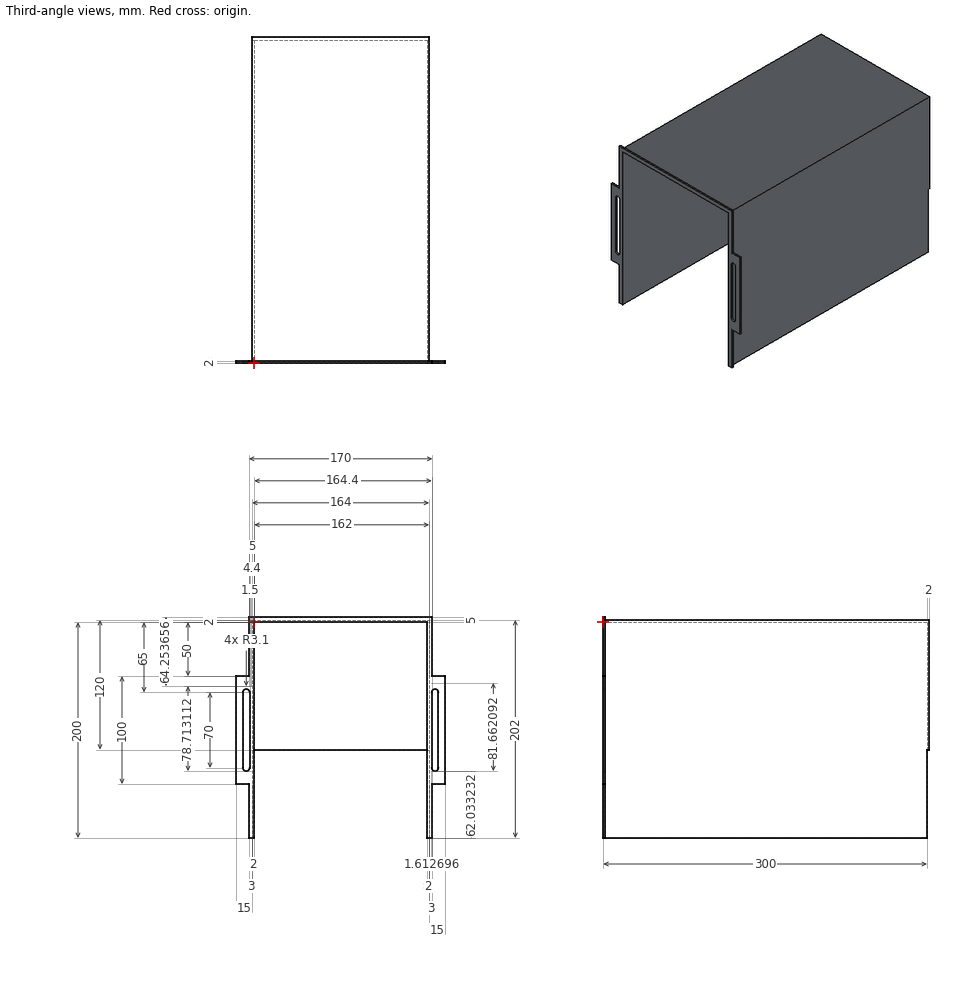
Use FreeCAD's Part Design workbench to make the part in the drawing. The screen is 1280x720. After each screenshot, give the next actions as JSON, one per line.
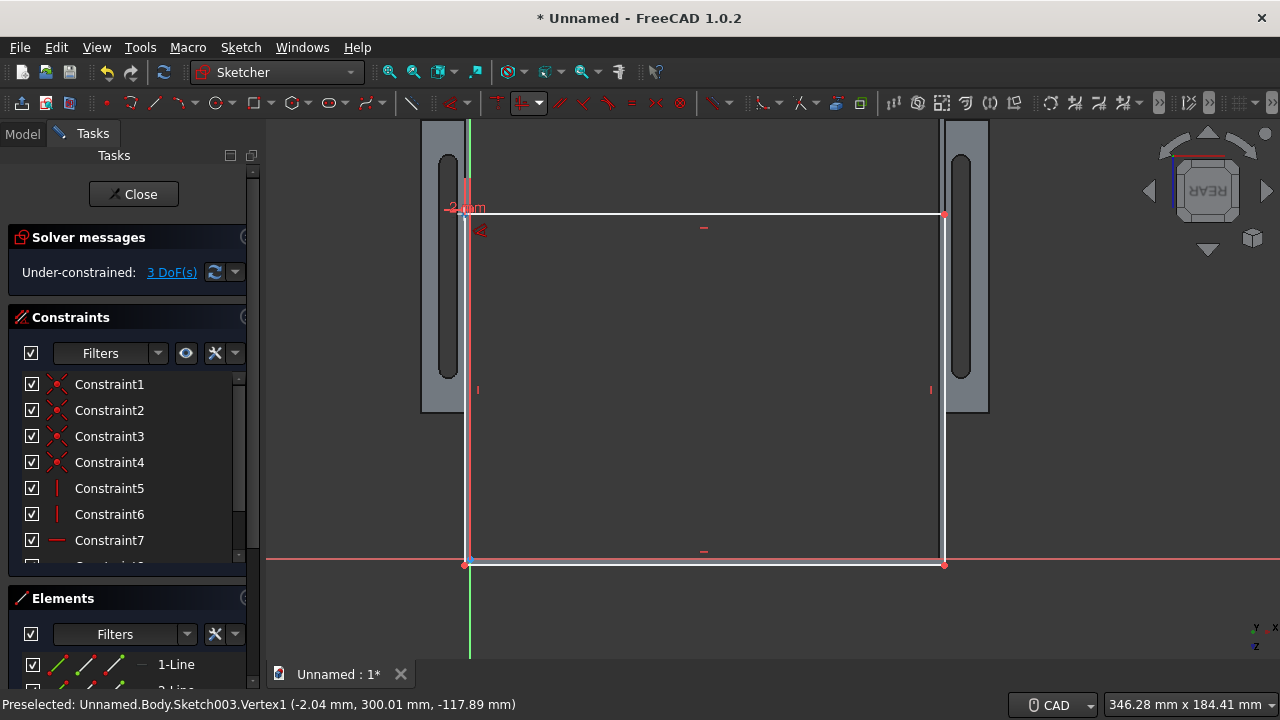
{"action": "scroll", "coordinate": [465, 565], "scroll_direction": "up", "scroll_amount": 10}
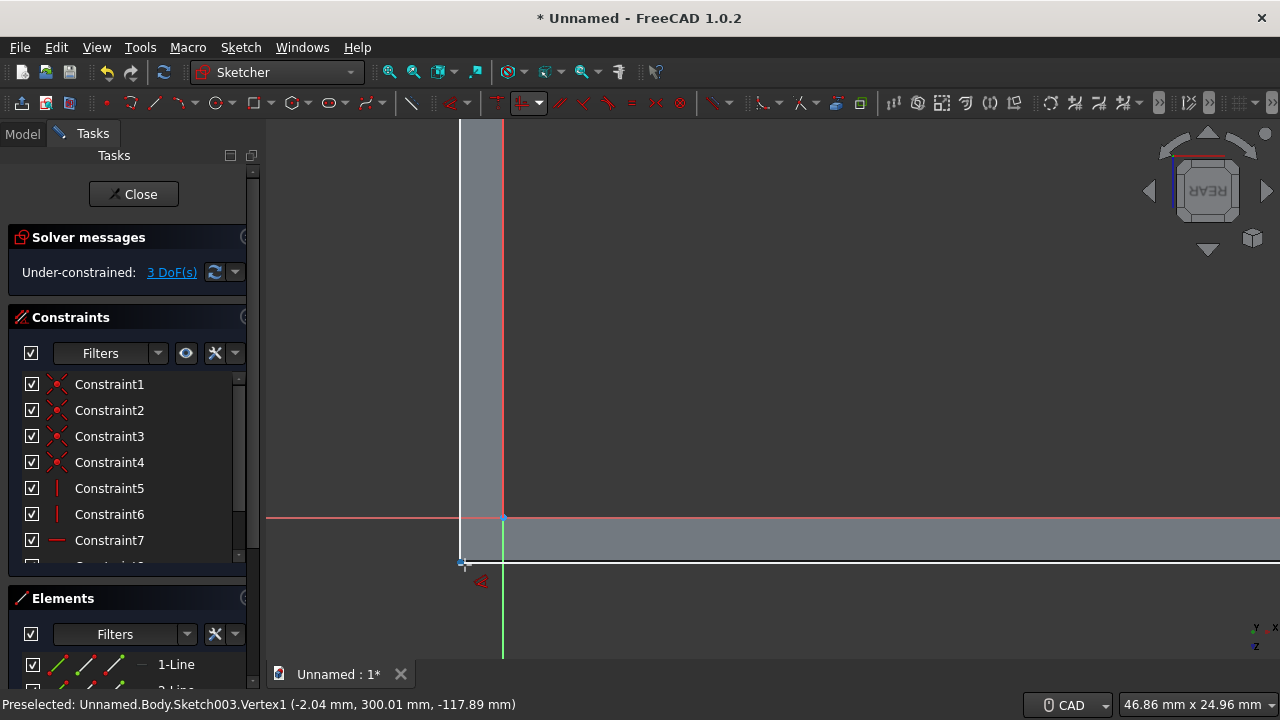
{"action": "left_click", "coordinate": [460, 563]}
{"action": "left_click", "coordinate": [426, 540]}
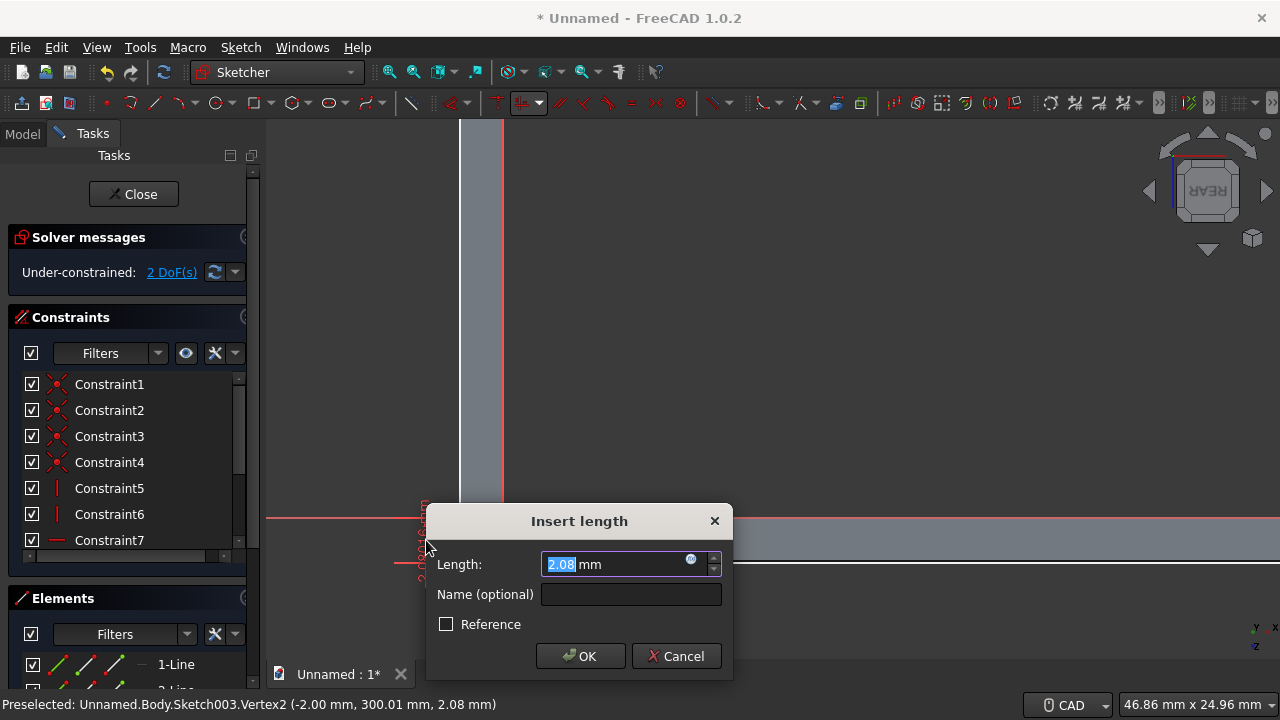
{"action": "type", "text": "2"}
{"action": "key", "text": "Return"}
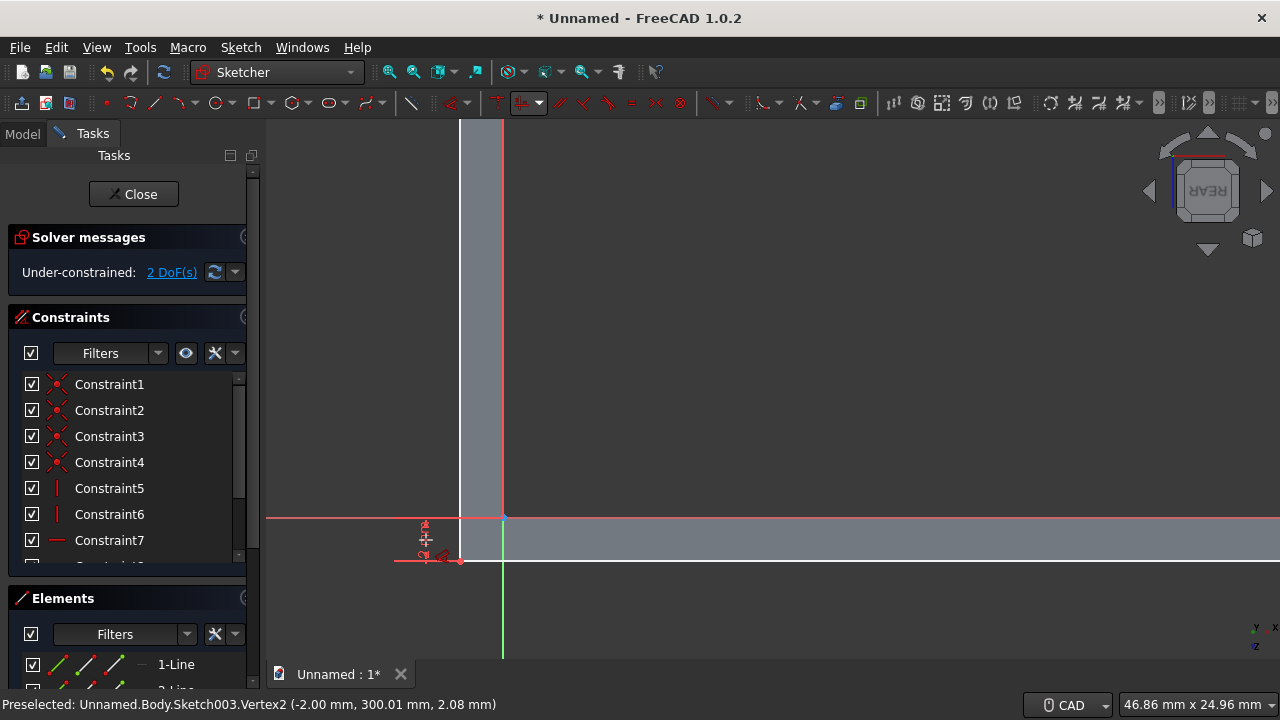
{"action": "scroll", "coordinate": [465, 565], "scroll_direction": "down", "scroll_amount": 10}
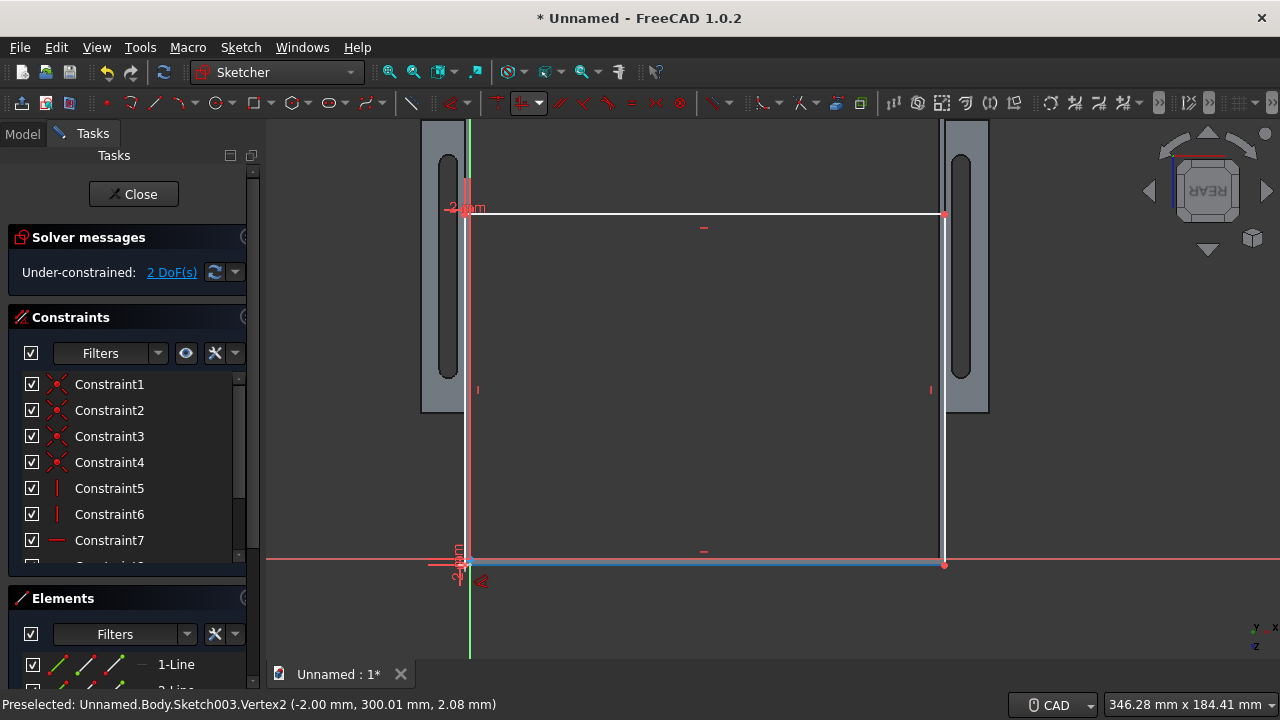
{"action": "scroll", "coordinate": [465, 319], "scroll_direction": "up", "scroll_amount": 5}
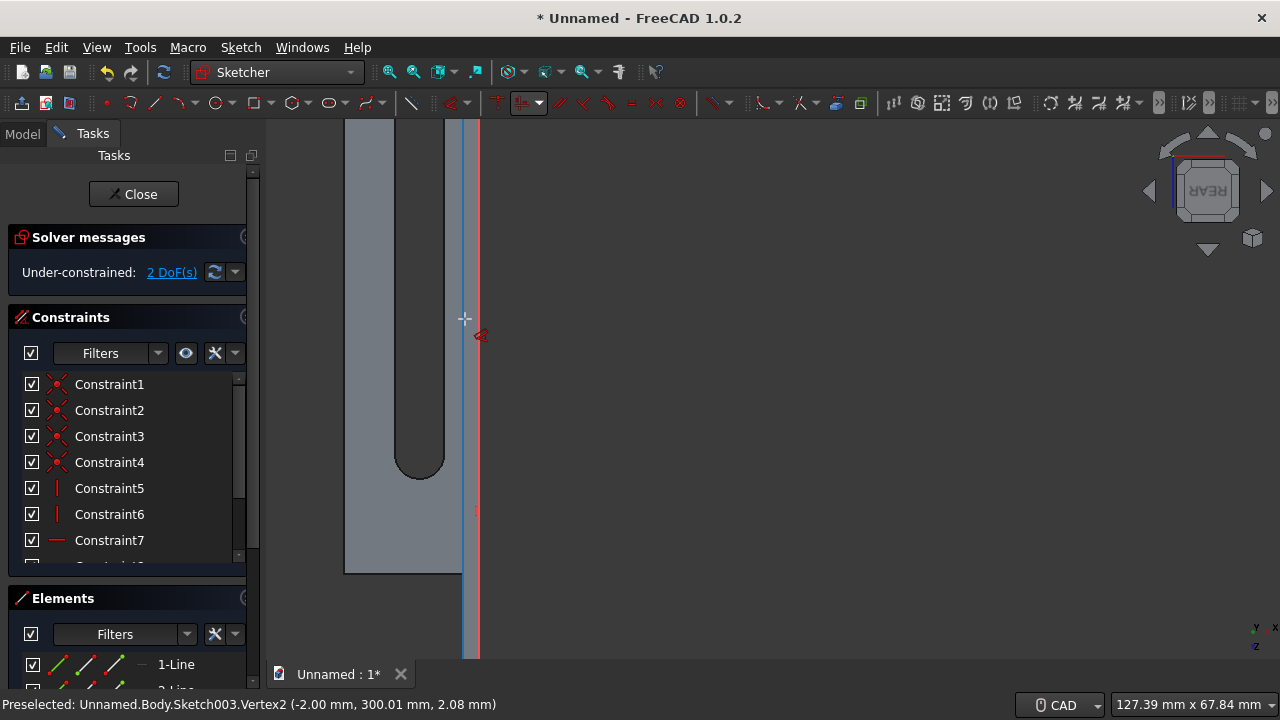
{"action": "left_click", "coordinate": [463, 320]}
{"action": "left_click", "coordinate": [429, 389]}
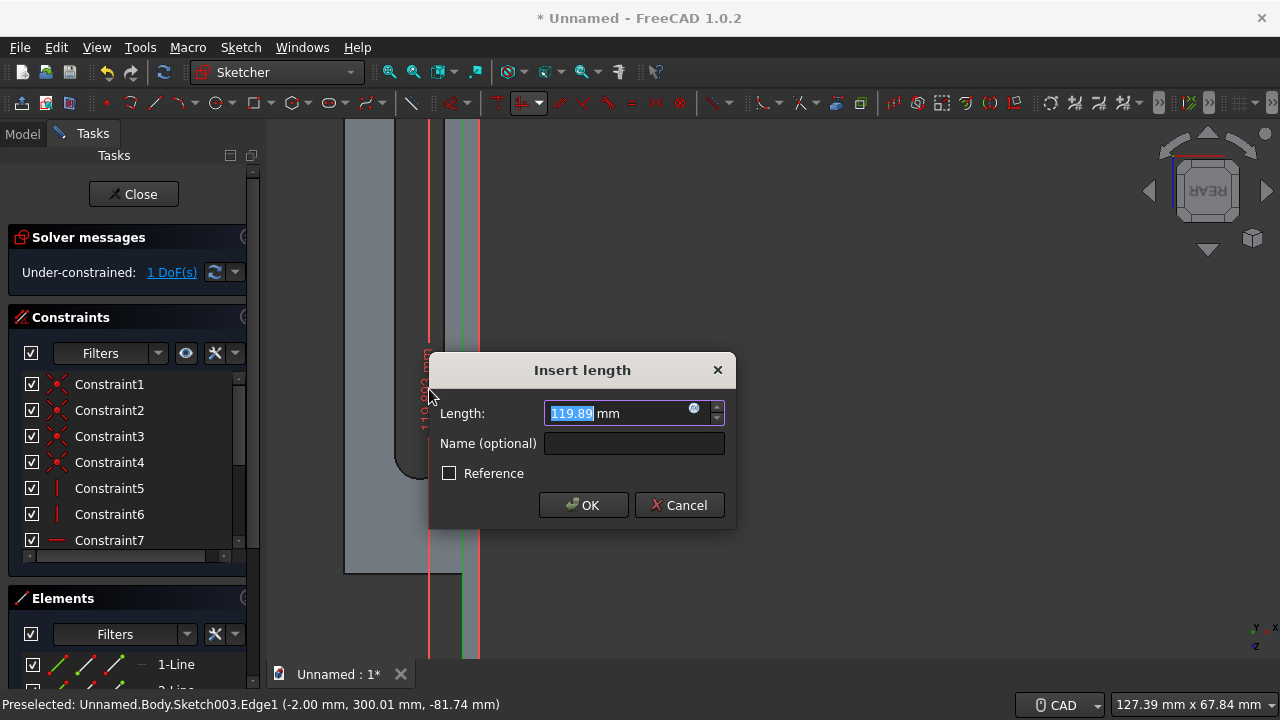
{"action": "type", "text": "120"}
{"action": "key", "text": "Return"}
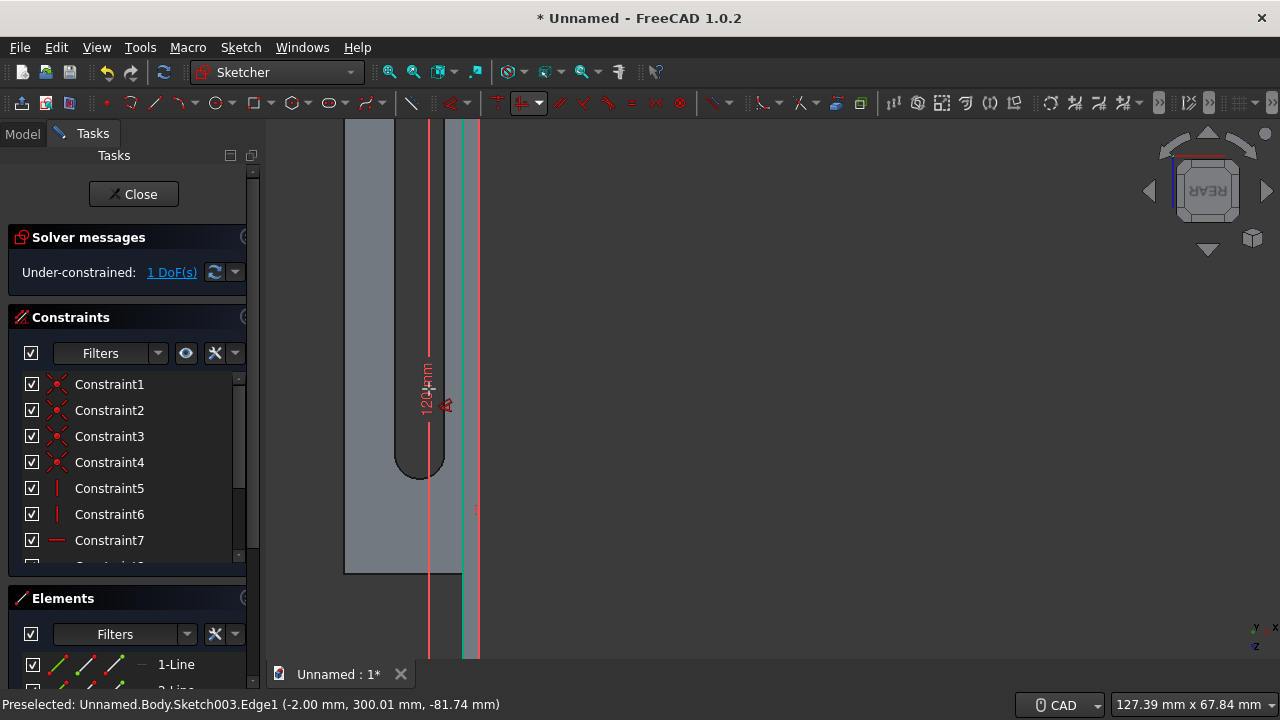
{"action": "scroll", "coordinate": [465, 319], "scroll_direction": "down", "scroll_amount": 5}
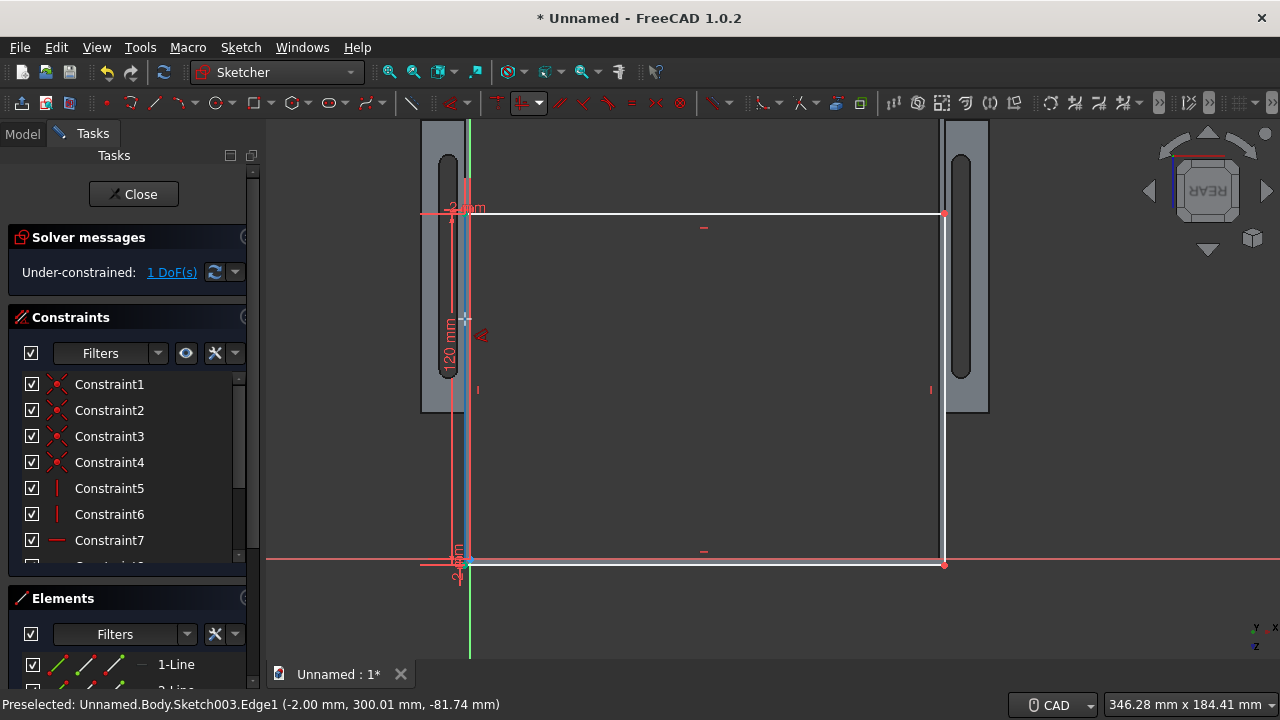
{"action": "scroll", "coordinate": [609, 565], "scroll_direction": "up", "scroll_amount": 5}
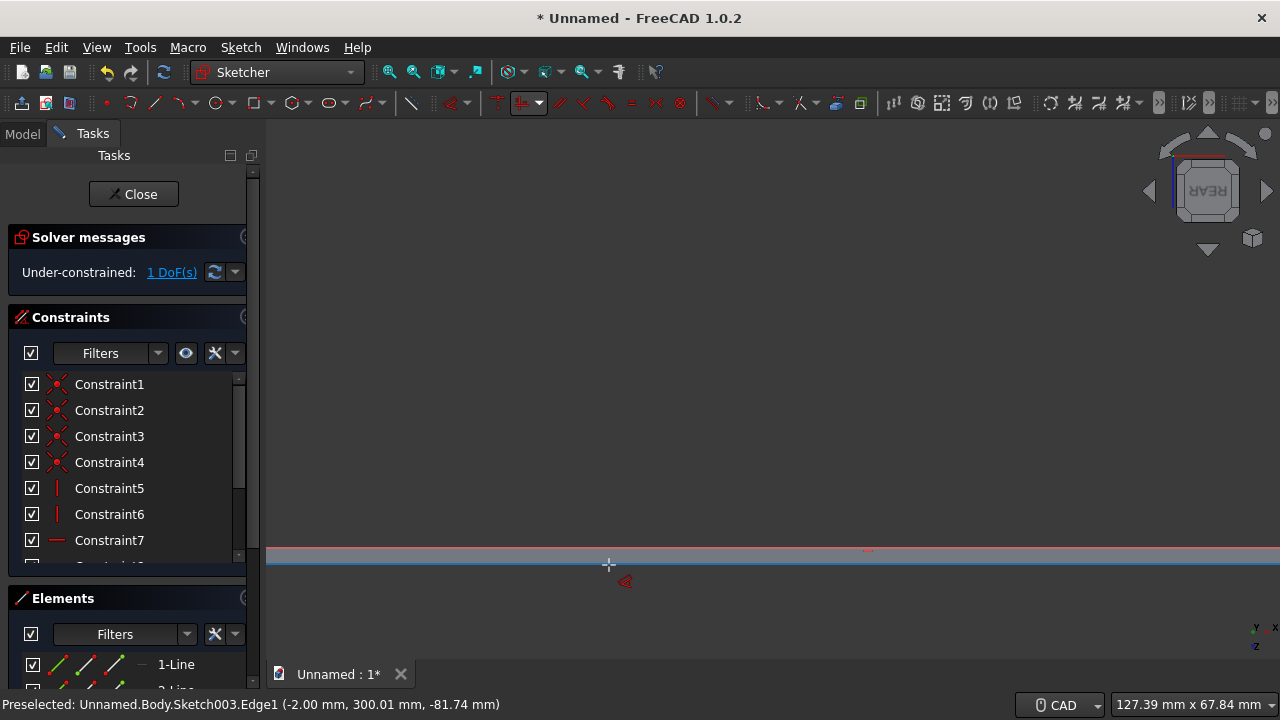
{"action": "left_click", "coordinate": [607, 564]}
{"action": "left_click", "coordinate": [704, 598]}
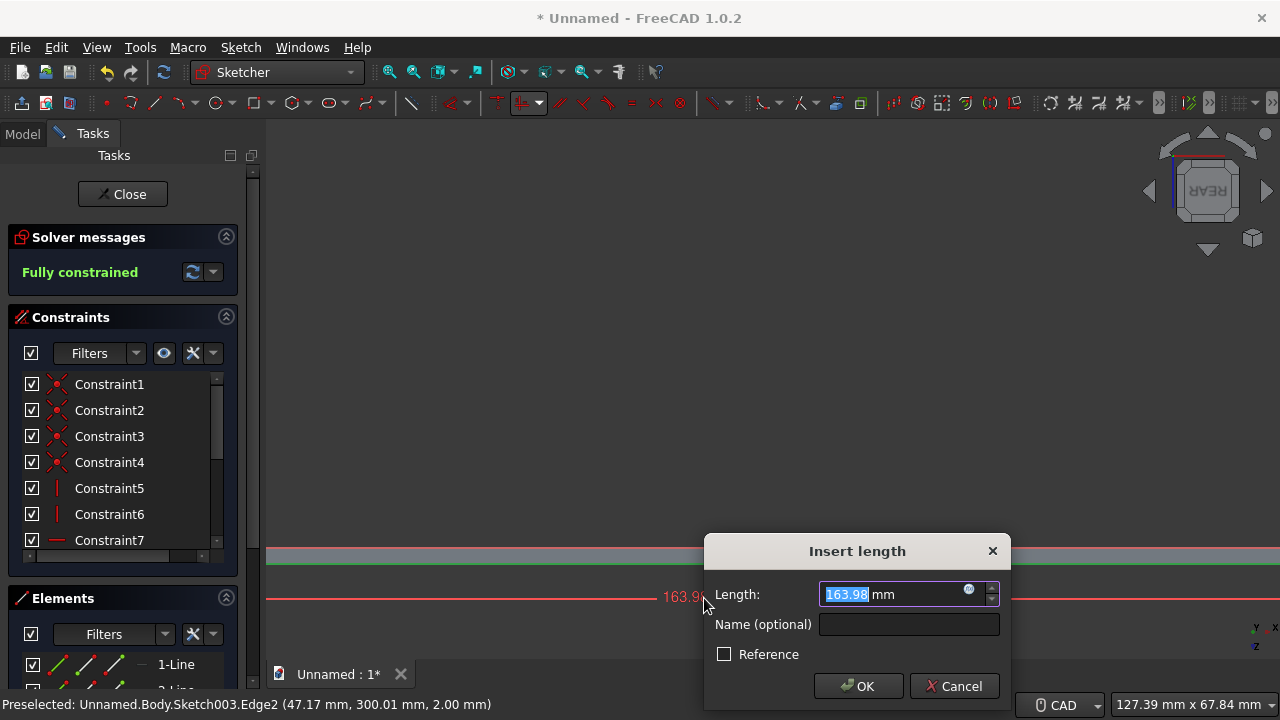
{"action": "type", "text": "164"}
{"action": "key", "text": "Return"}
{"action": "key", "text": "Escape"}